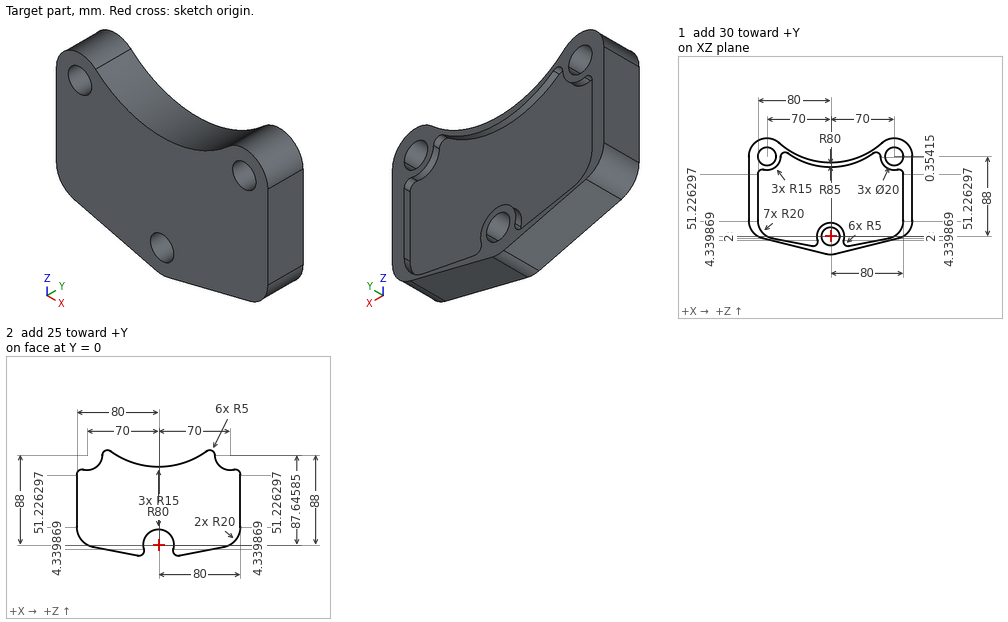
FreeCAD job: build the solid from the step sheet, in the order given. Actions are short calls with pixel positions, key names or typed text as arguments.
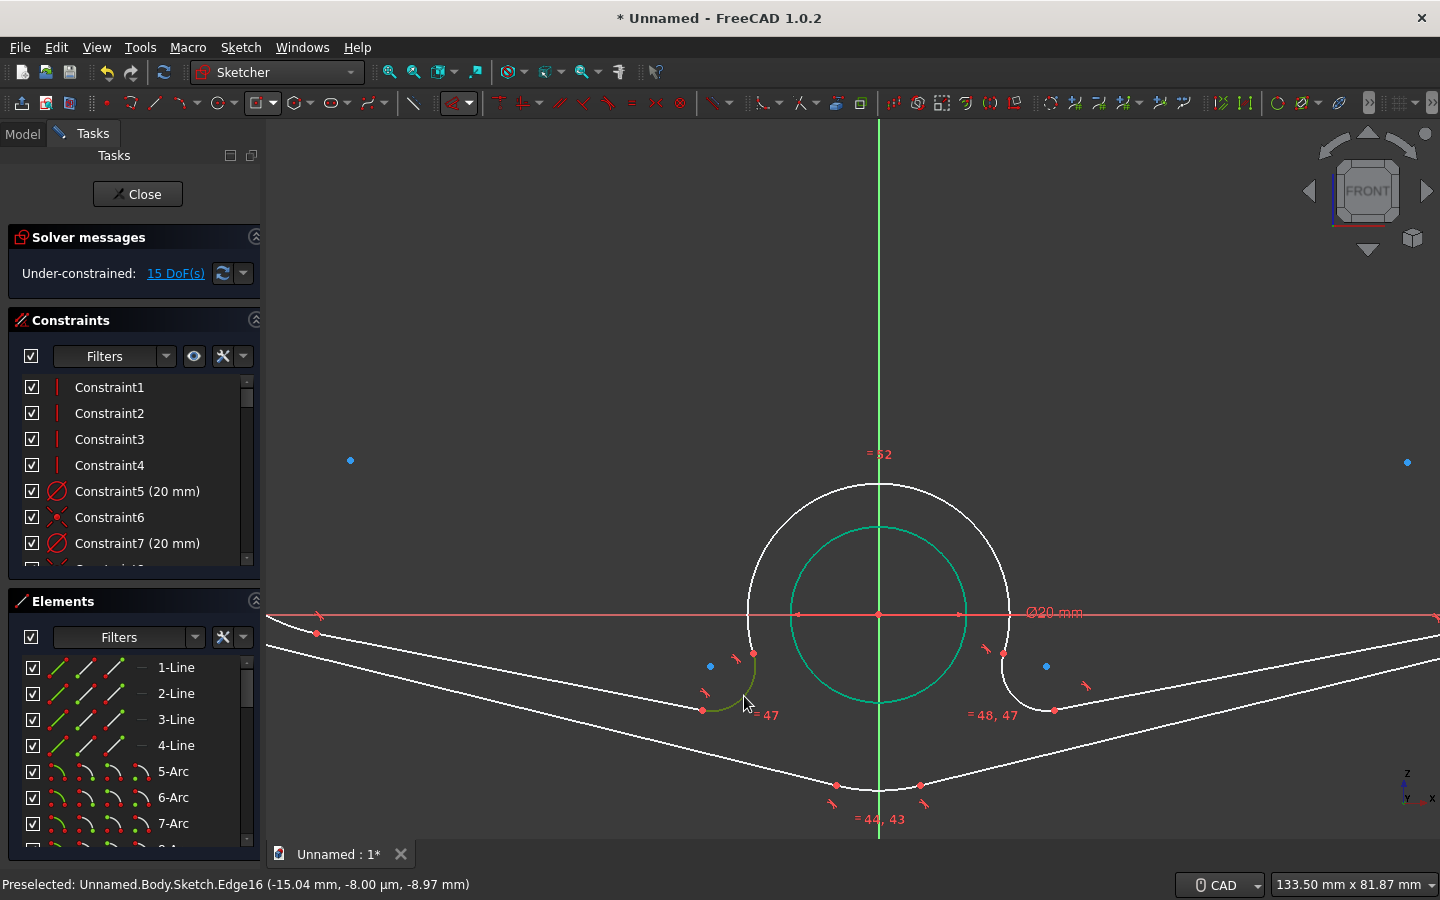
click(472, 104)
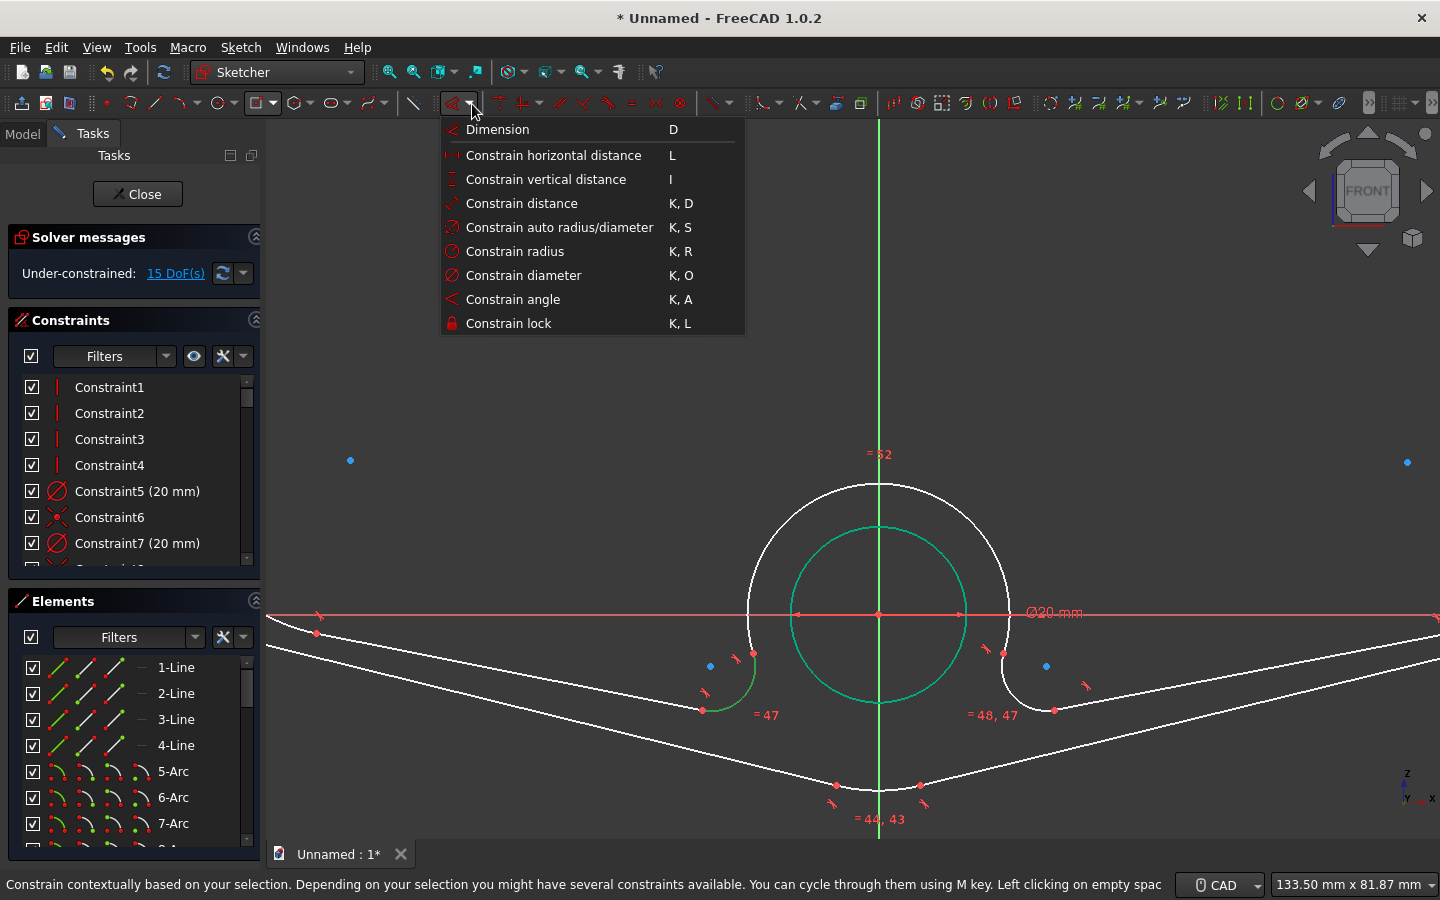
click(593, 251)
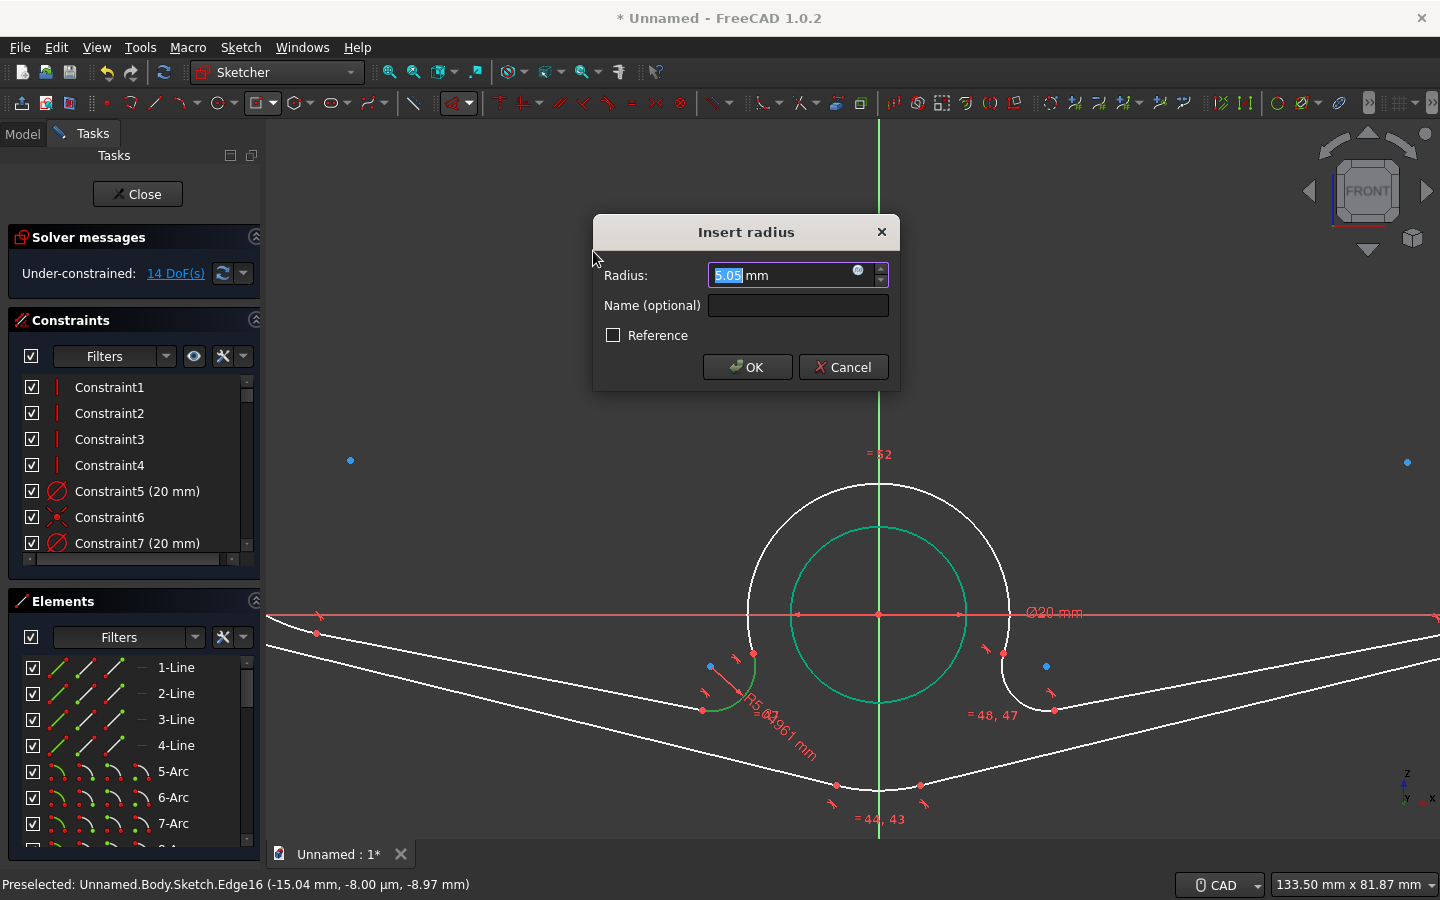
text(5)
key(Return)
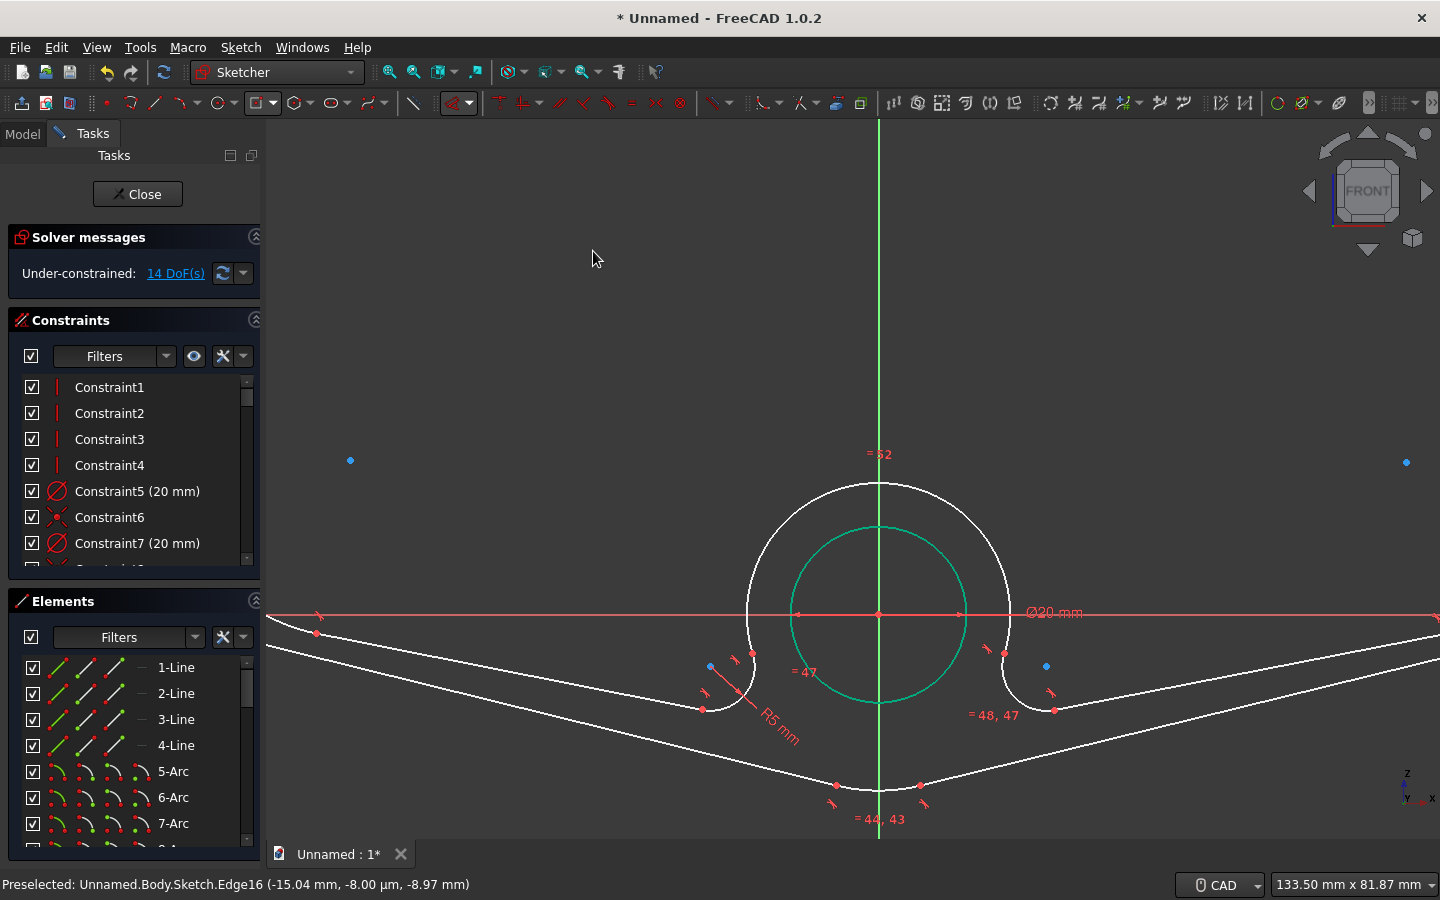
click(968, 518)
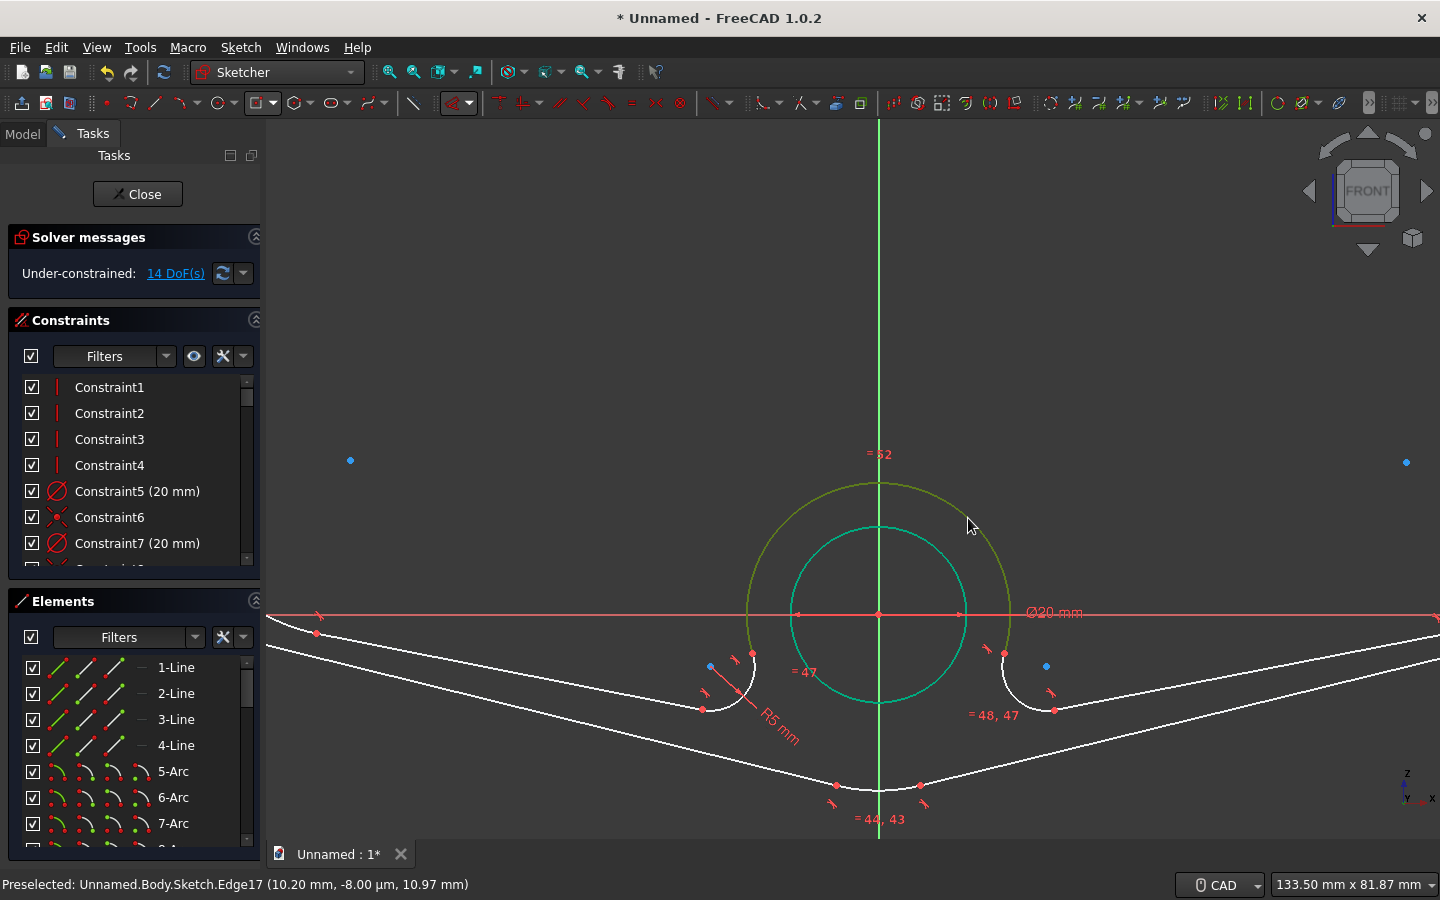
key(k)
key(r)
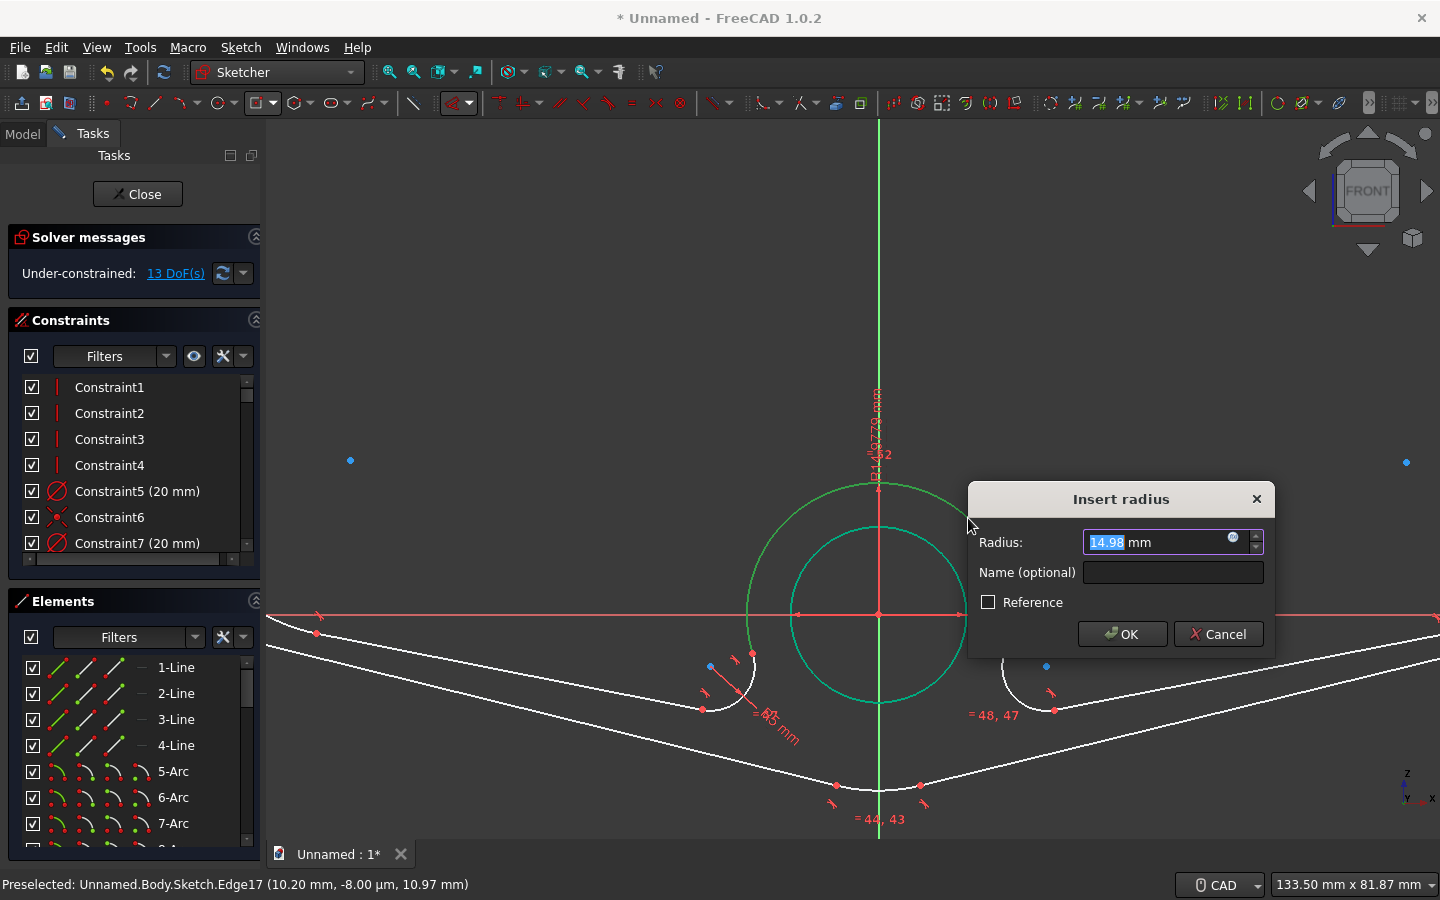
text(15)
key(Return)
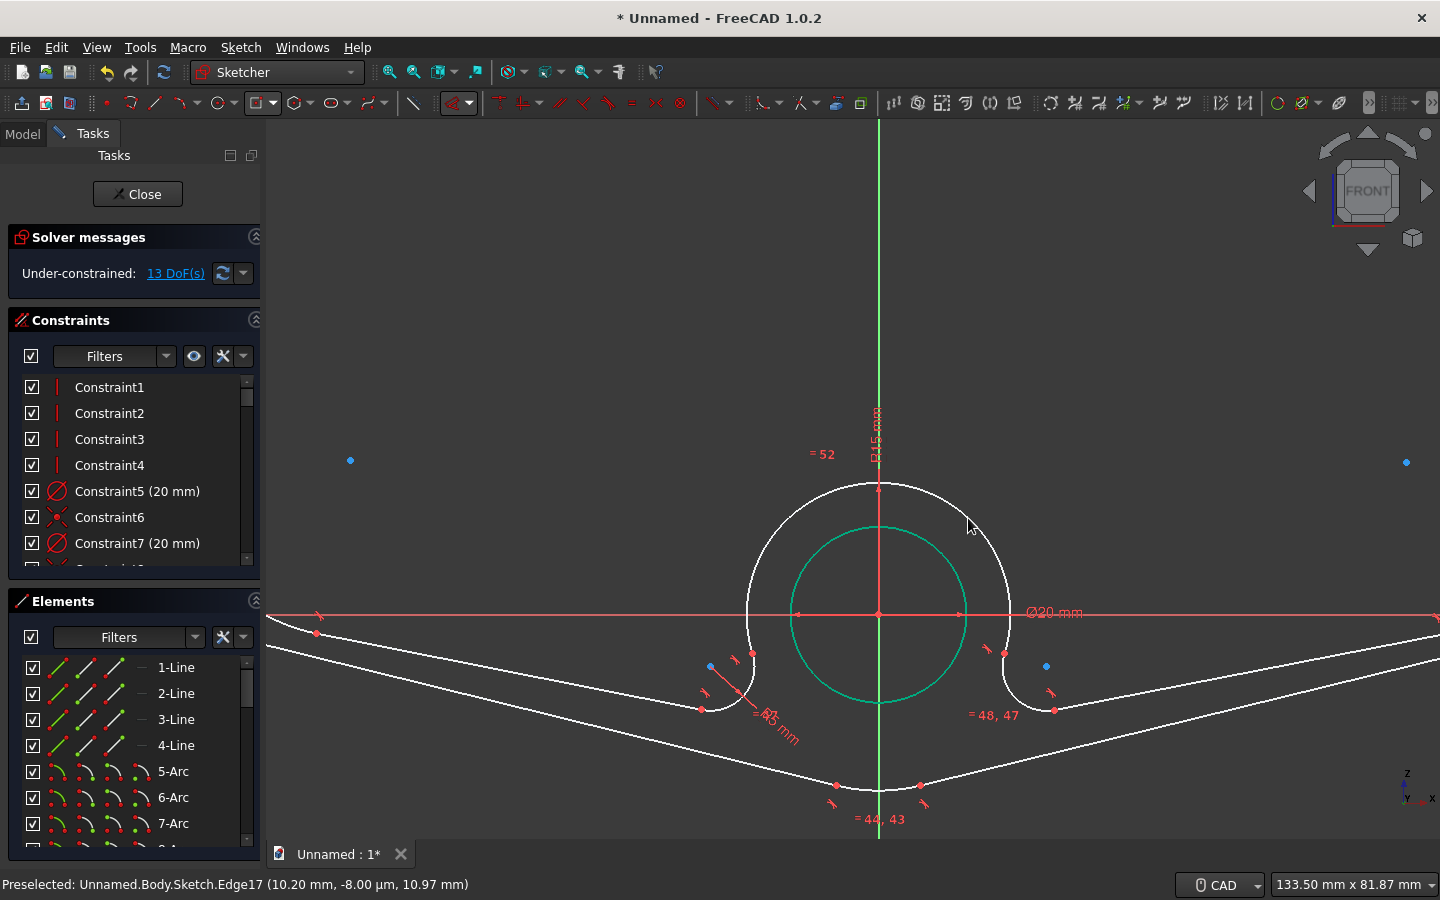
scroll(708, 678, down, 4)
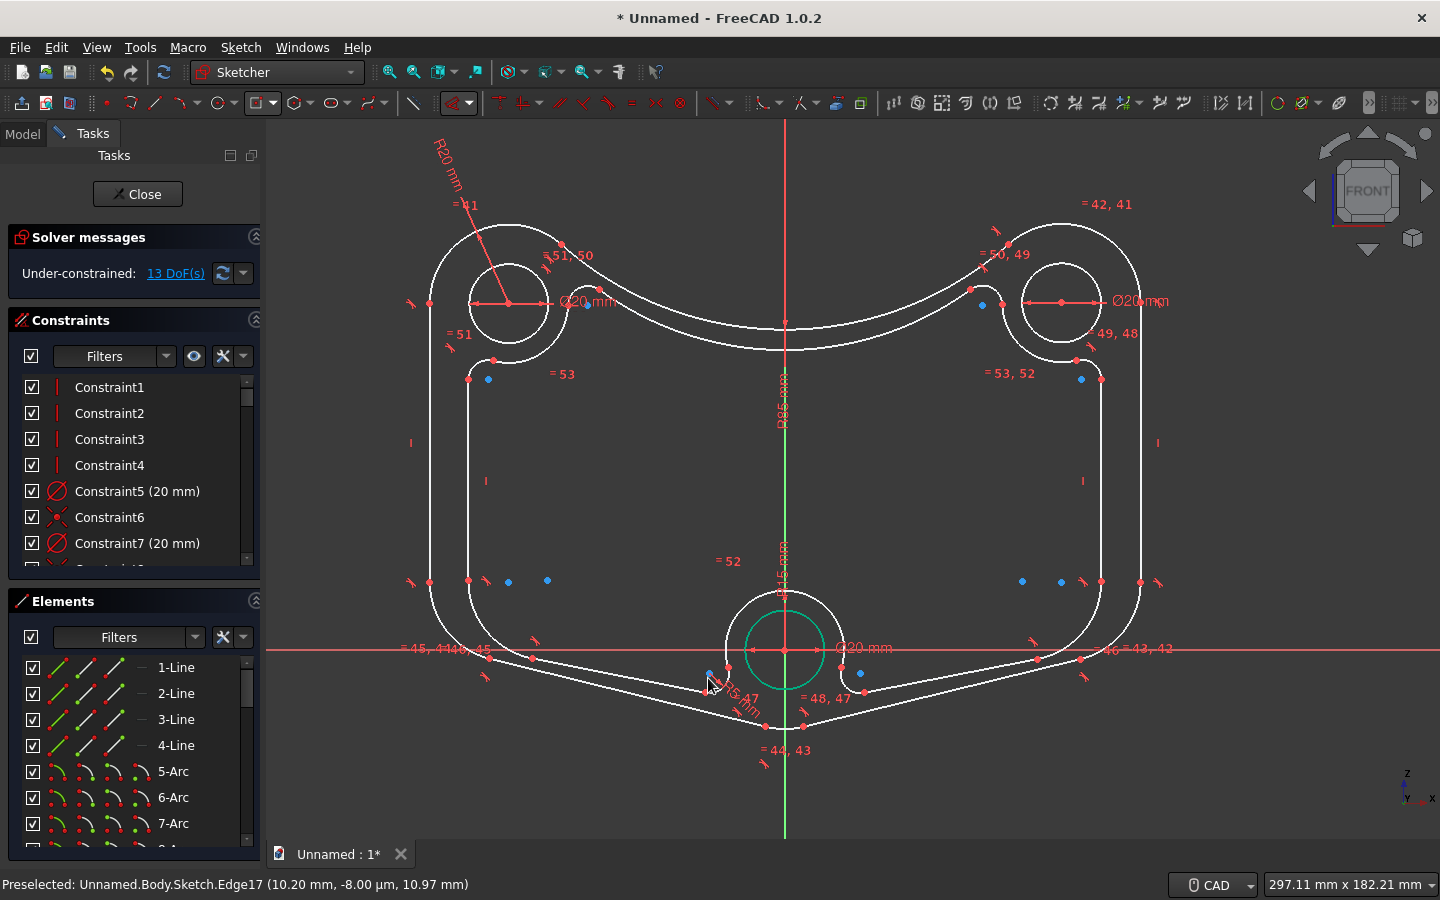
click(707, 340)